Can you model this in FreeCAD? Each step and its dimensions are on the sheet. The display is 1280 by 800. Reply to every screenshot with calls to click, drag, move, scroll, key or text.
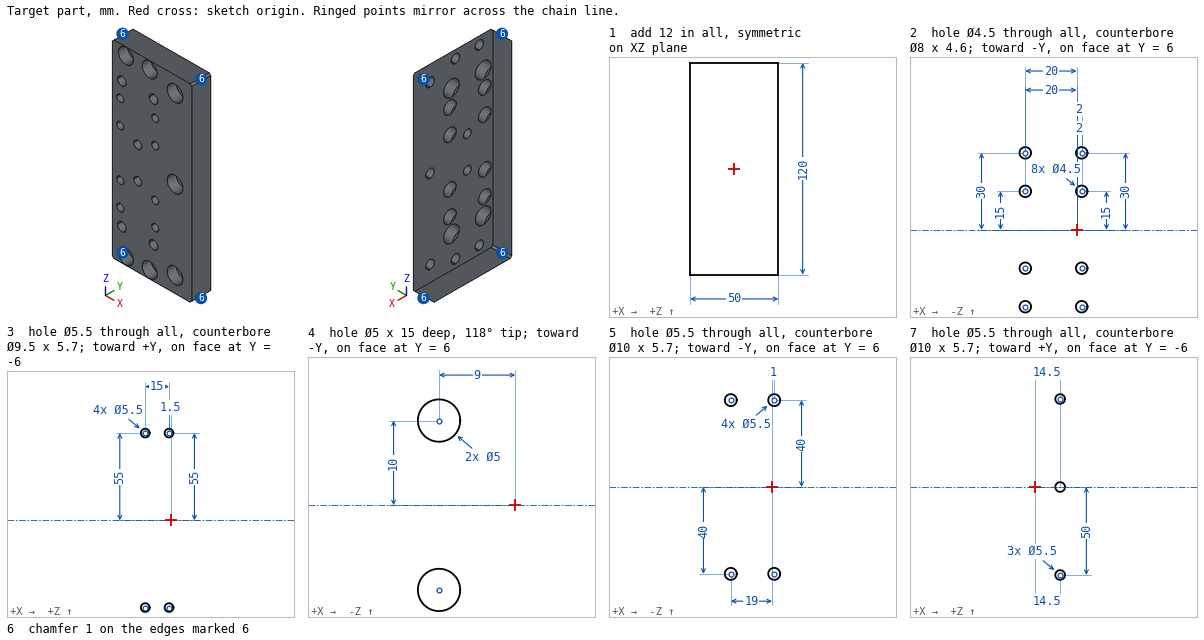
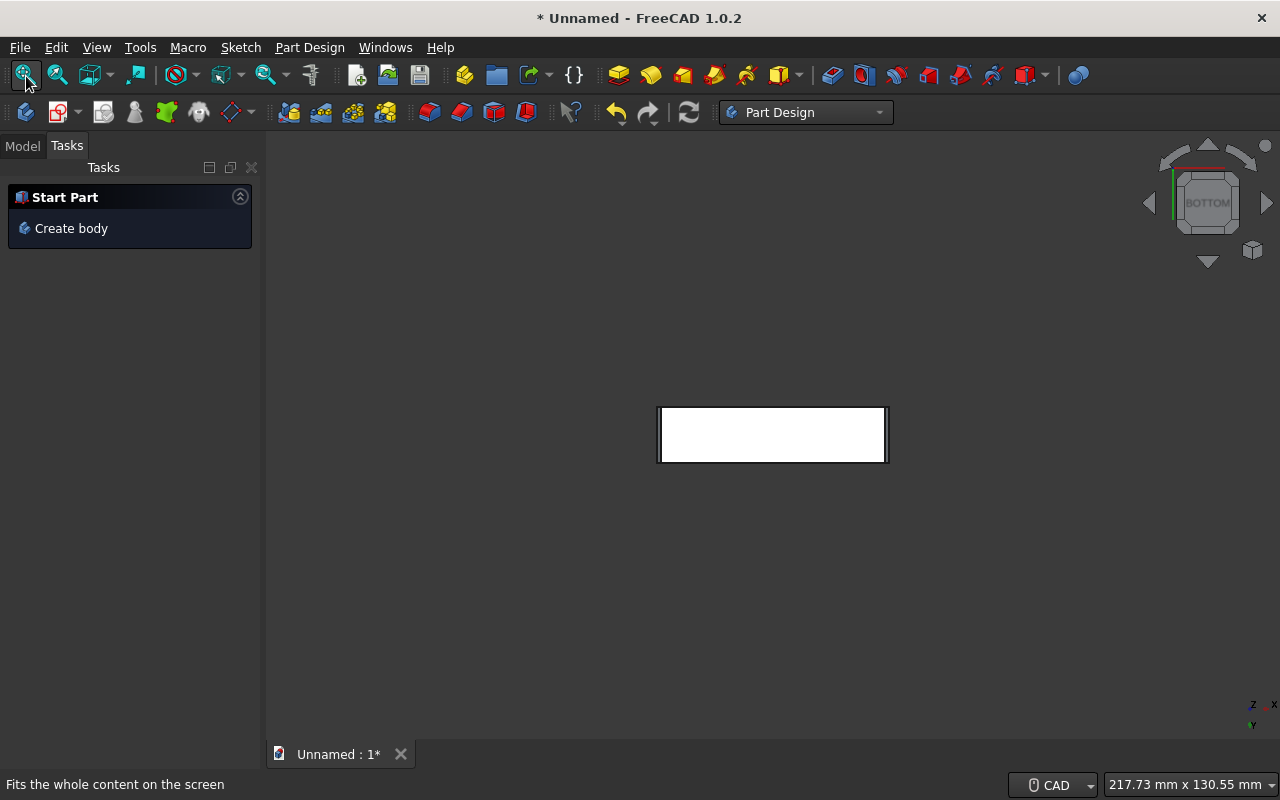
key(0)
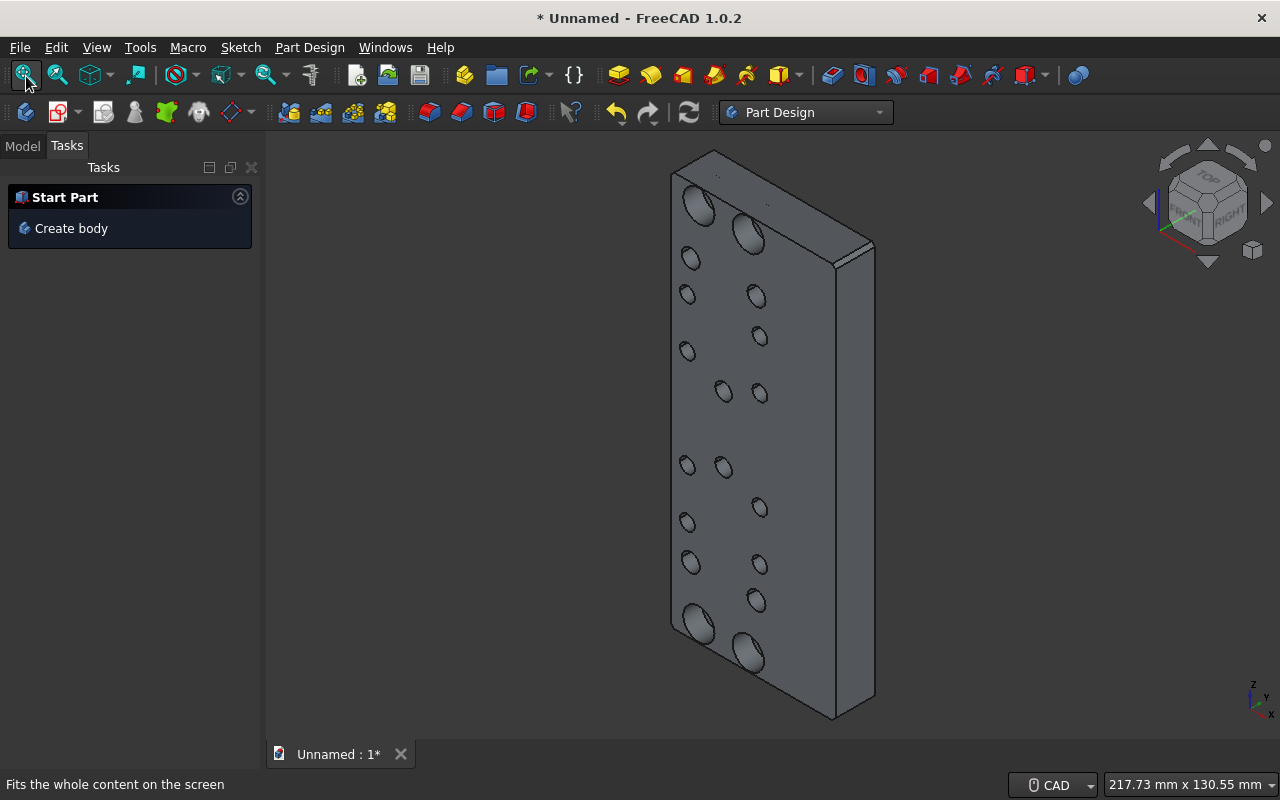
click(777, 459)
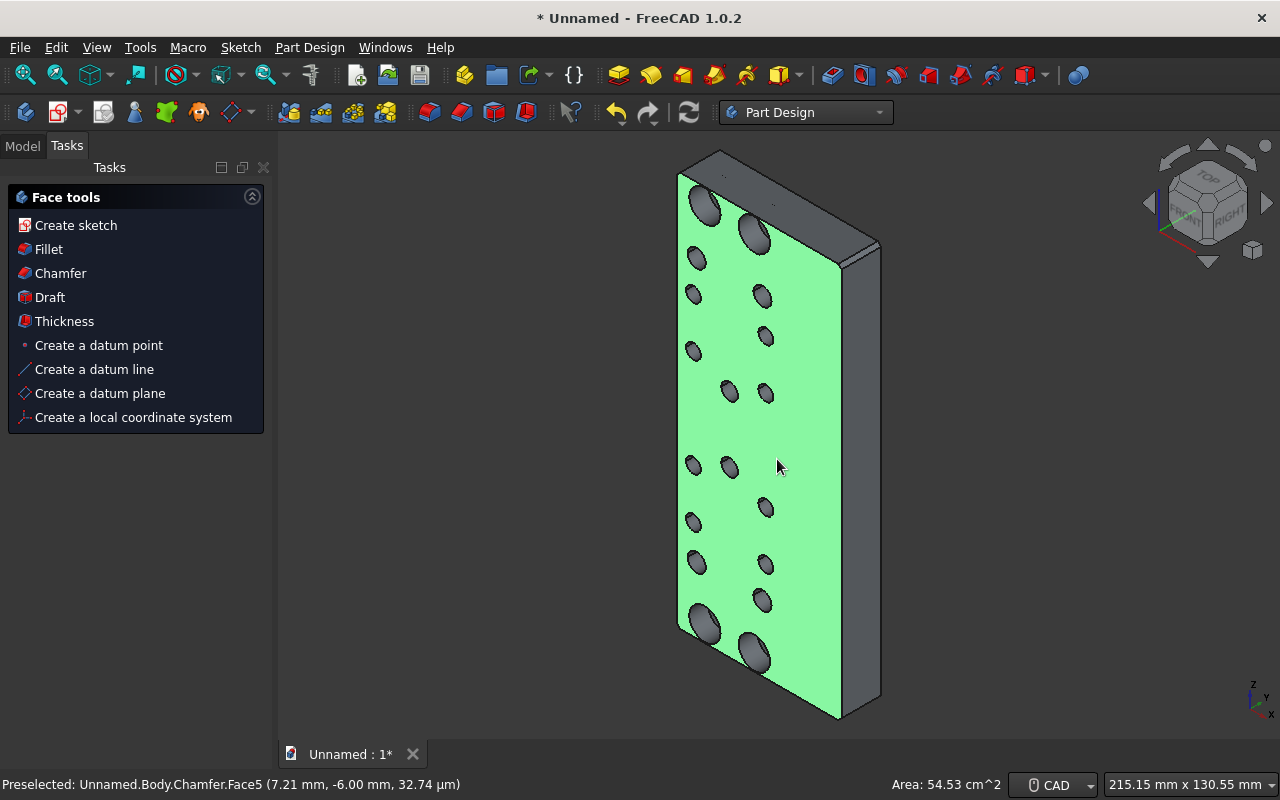
click(58, 112)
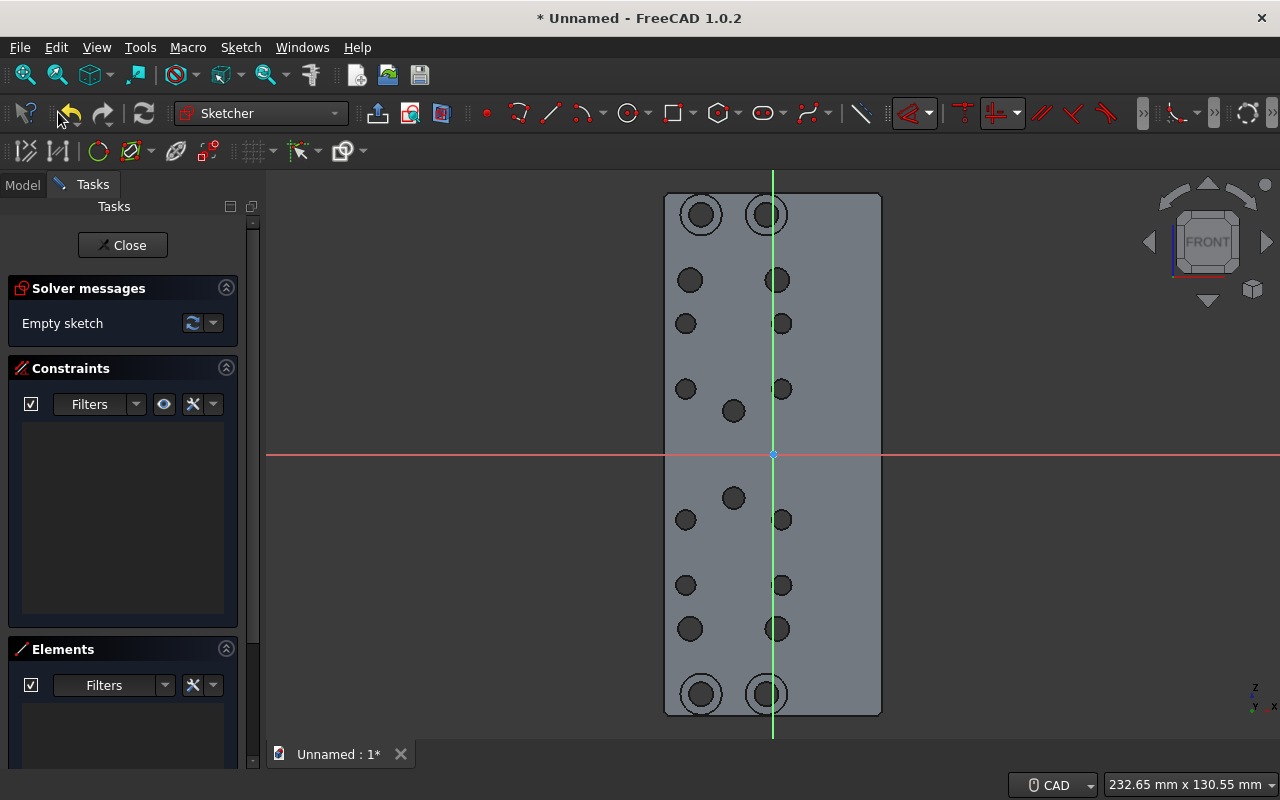
click(628, 114)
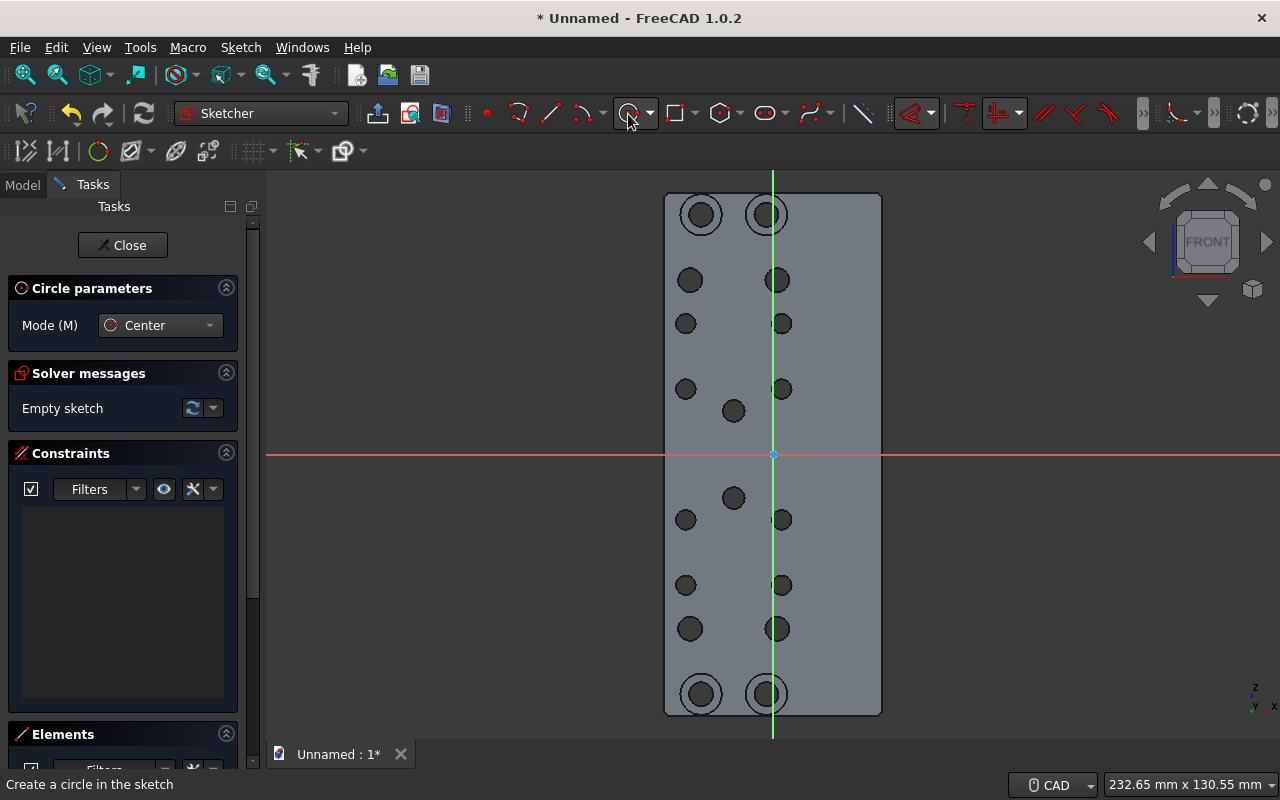
scroll(836, 672, up, 4)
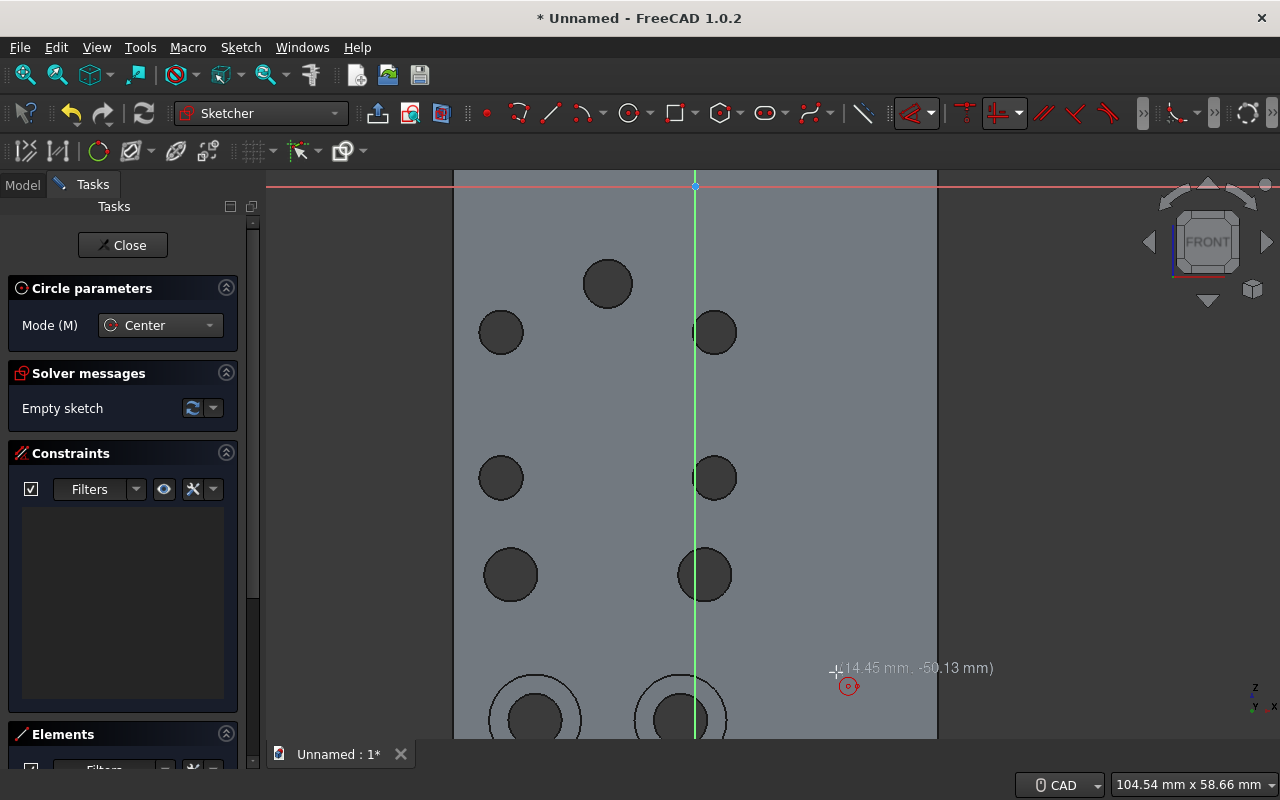
click(836, 672)
move(855, 653)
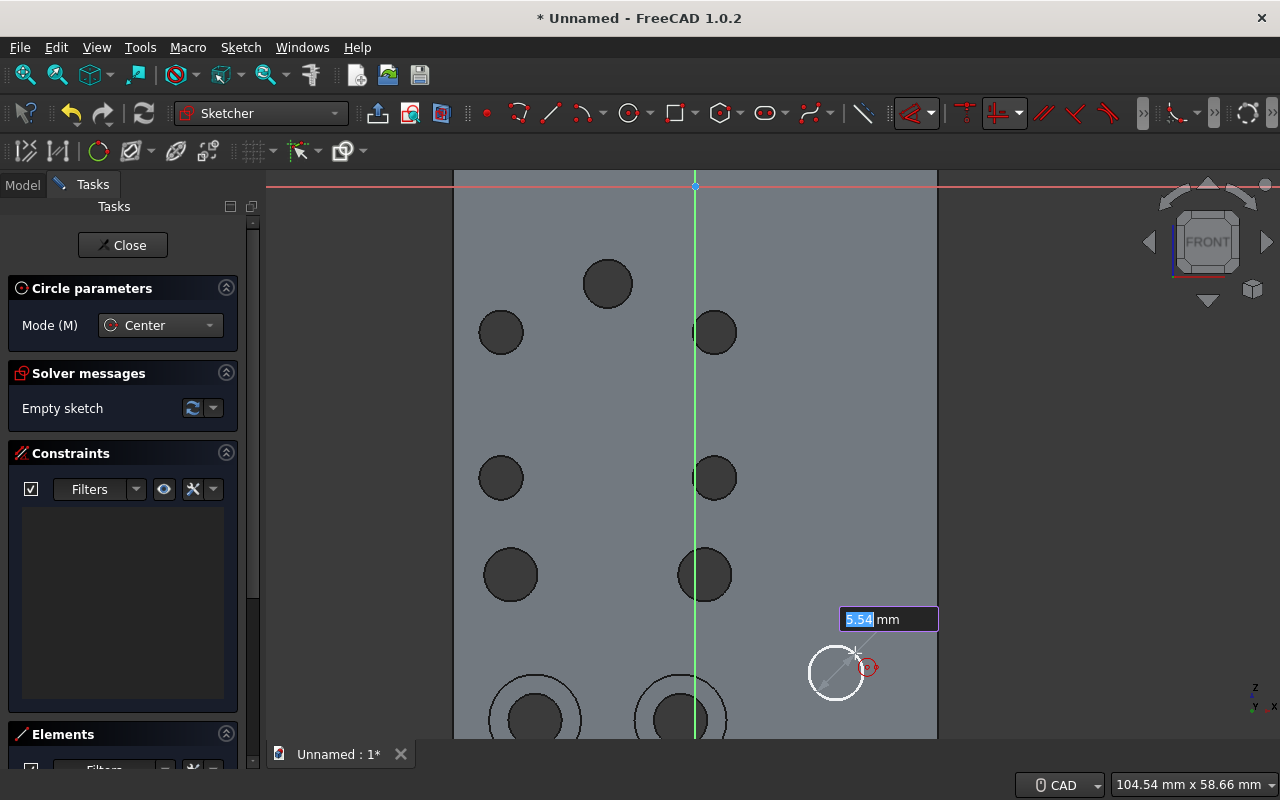
text(5.5)
key(Return)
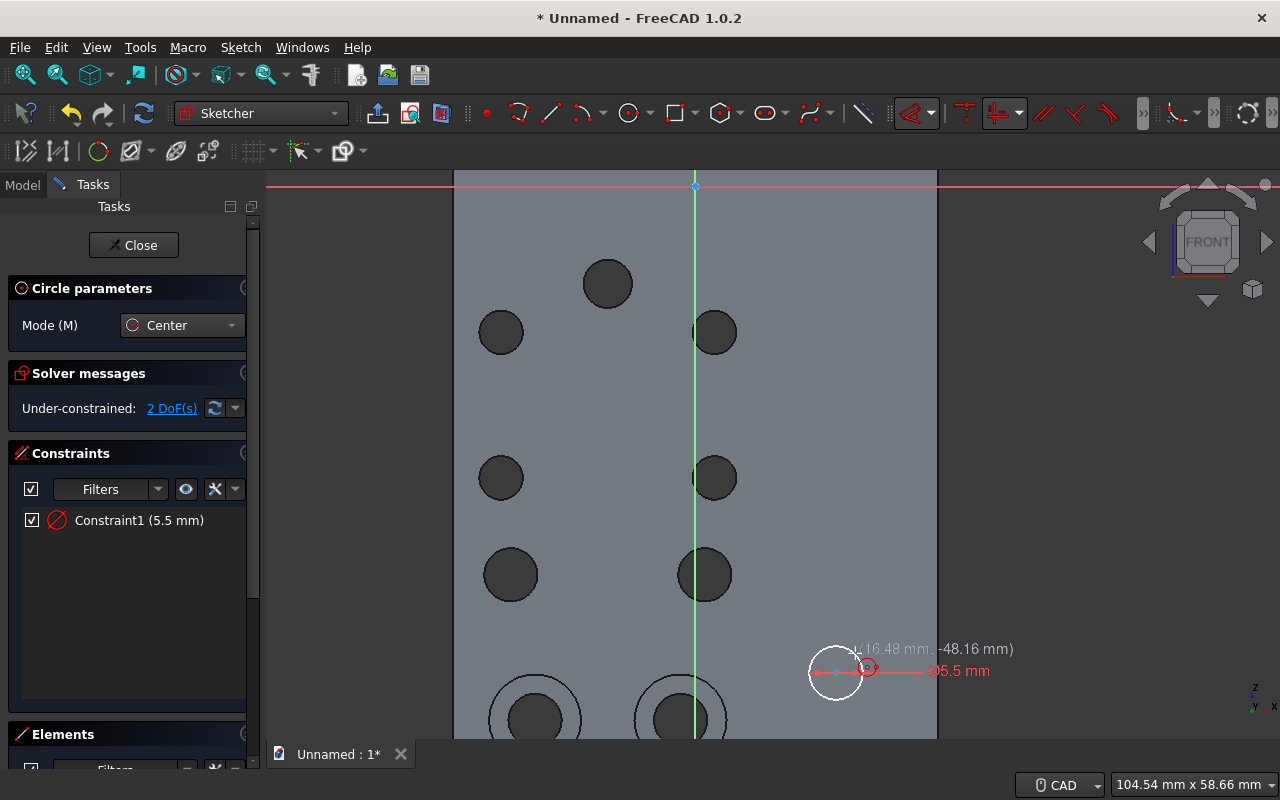
scroll(661, 610, down, 5)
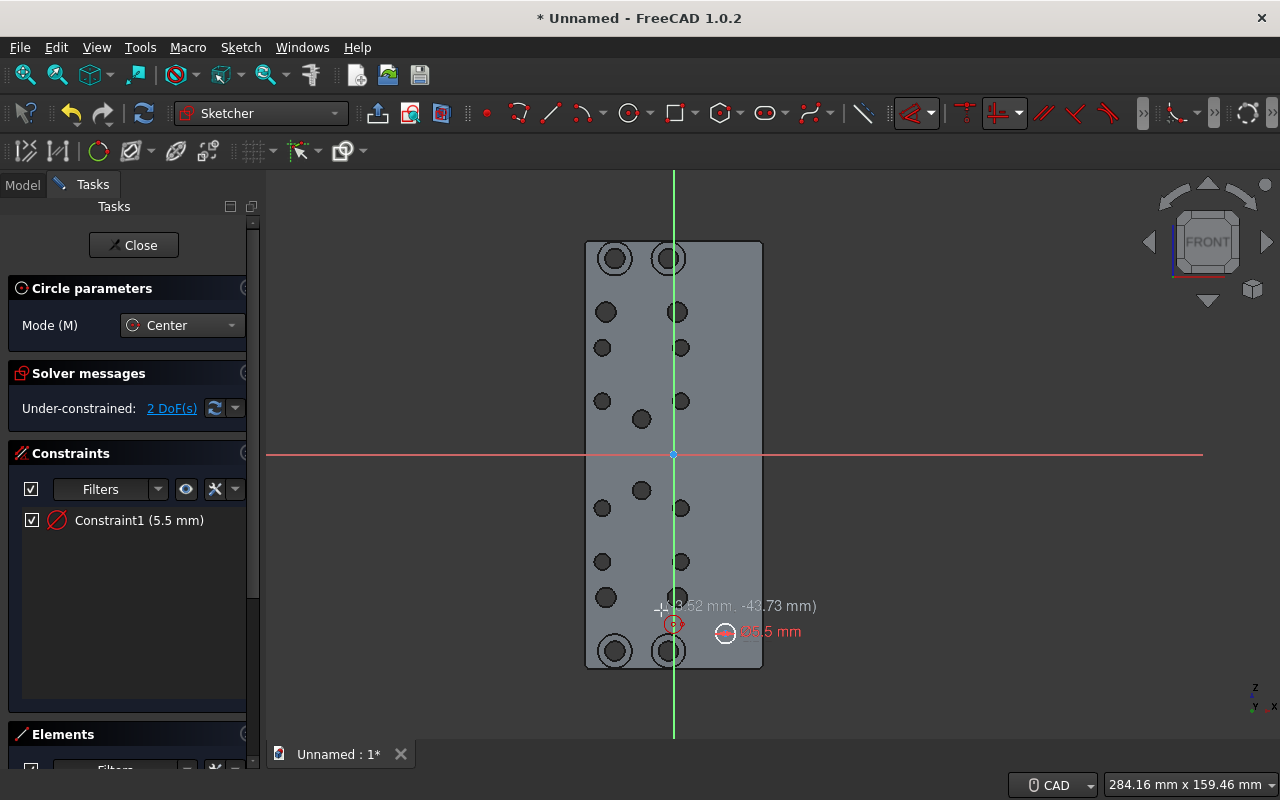
scroll(726, 455, up, 5)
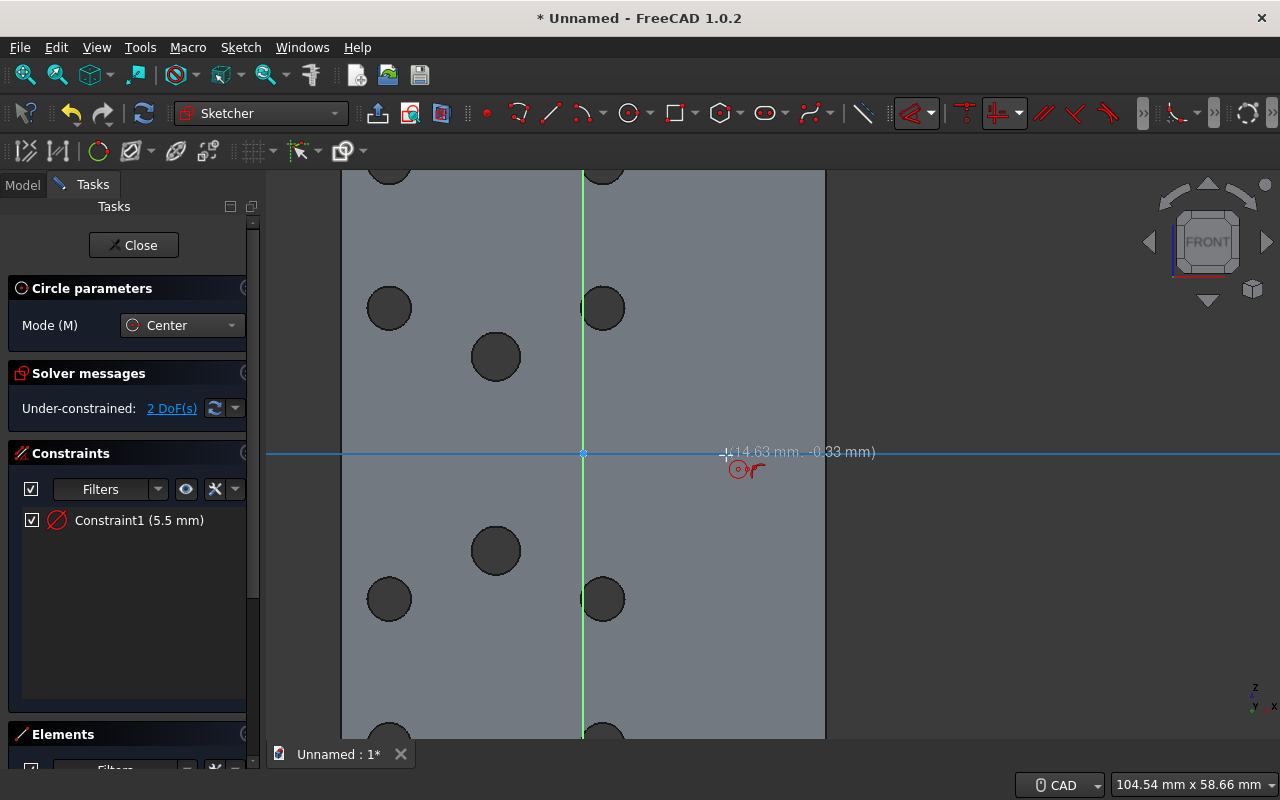
click(724, 454)
move(743, 435)